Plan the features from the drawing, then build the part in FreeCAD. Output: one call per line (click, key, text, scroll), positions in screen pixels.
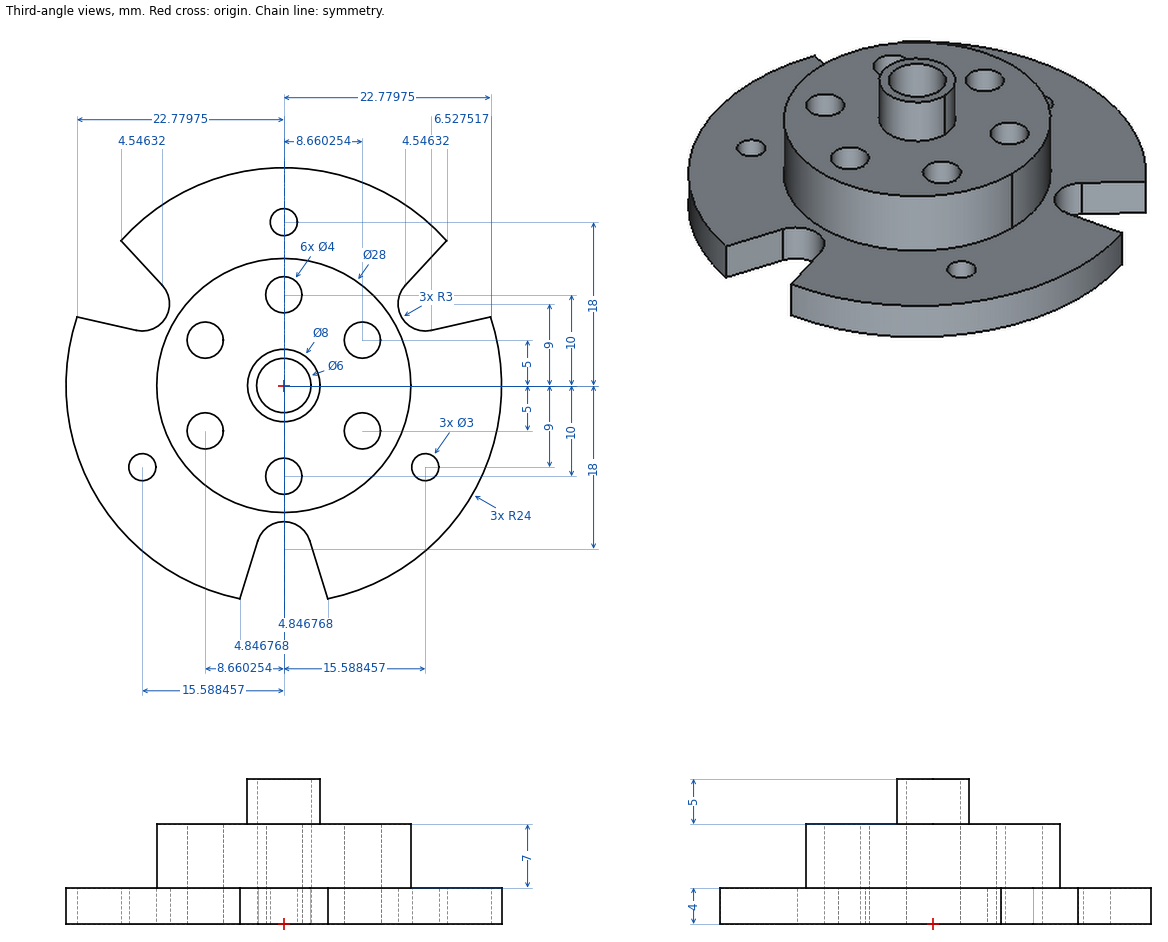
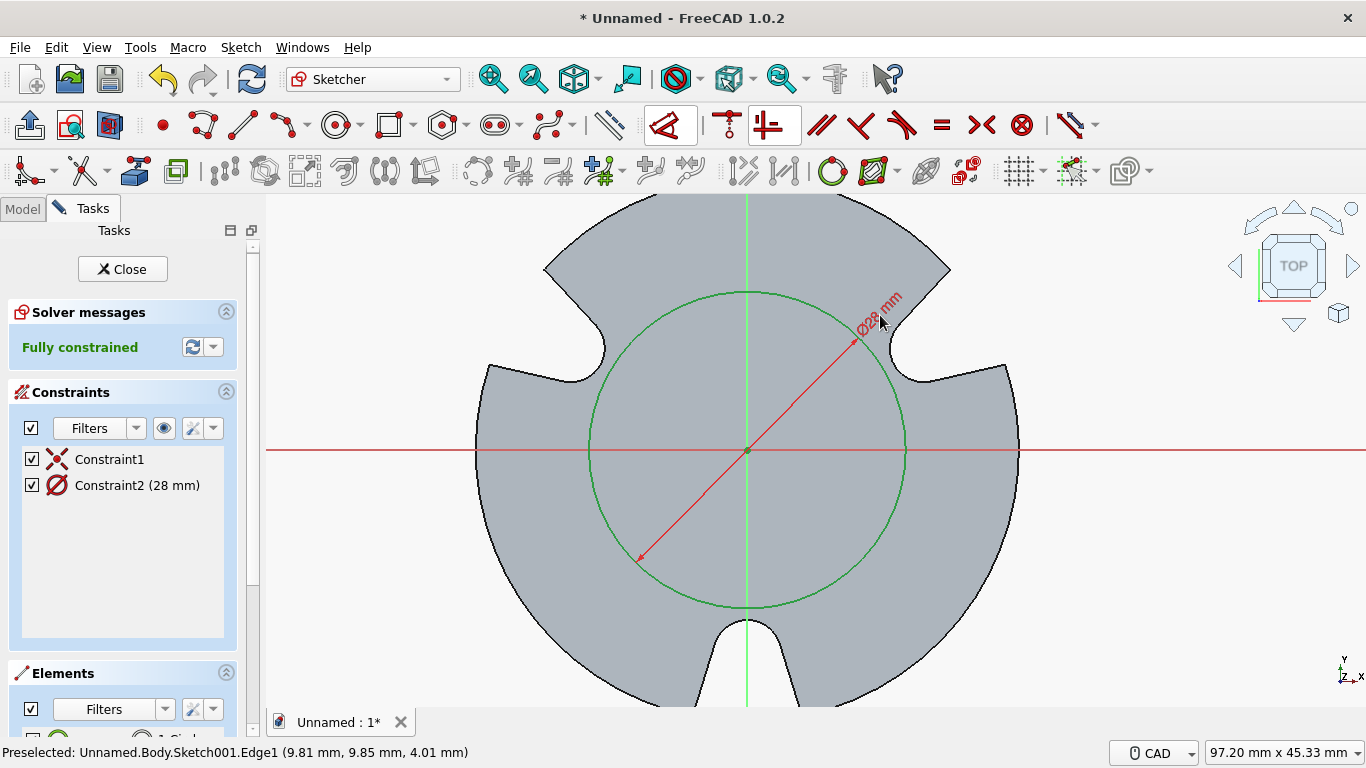
click(123, 269)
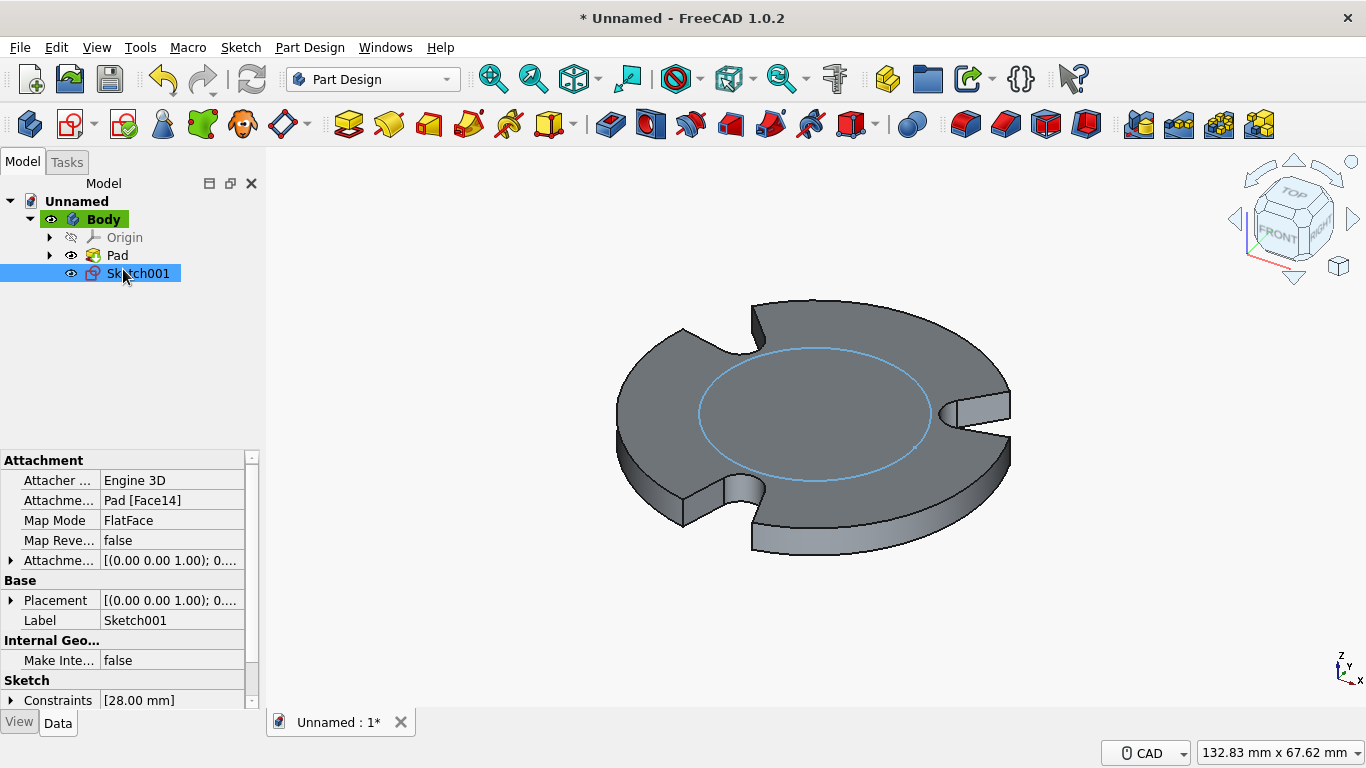
click(350, 124)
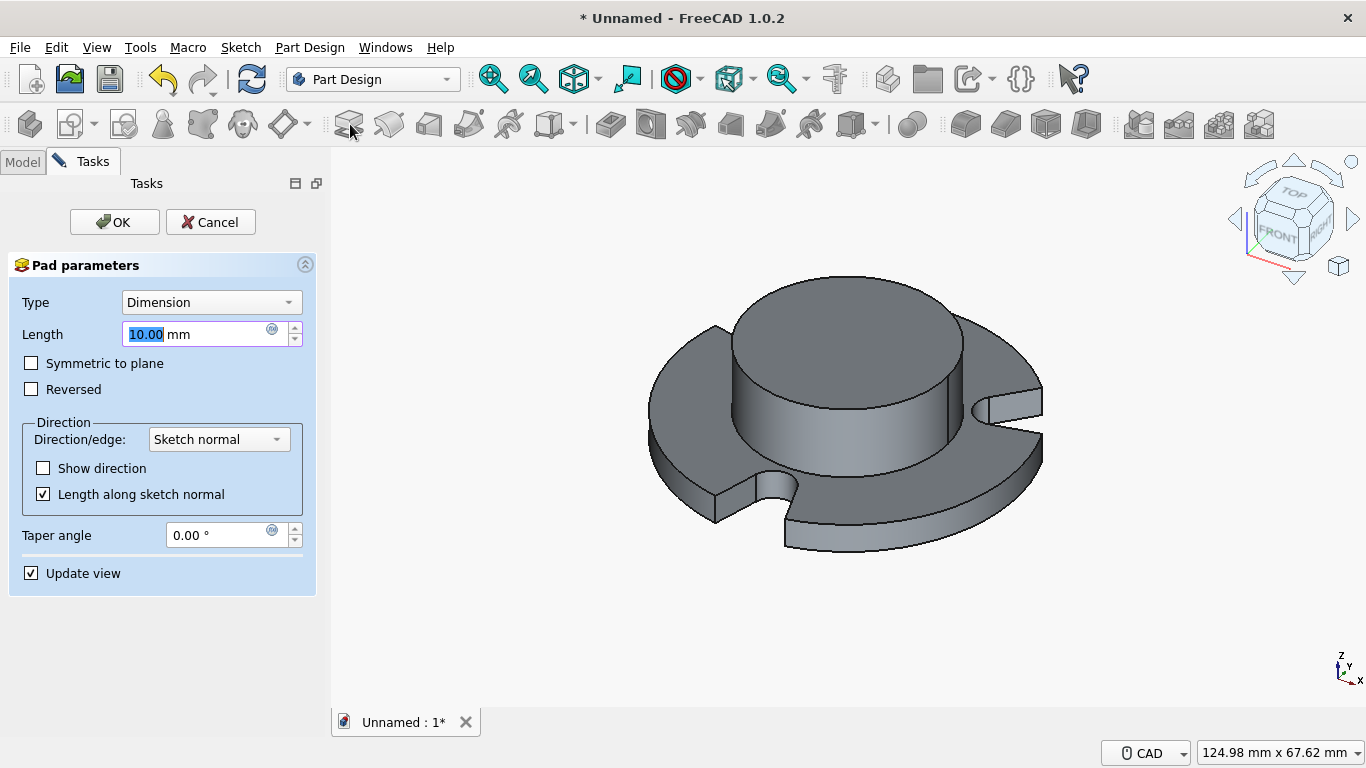
text(7)
key(Tab)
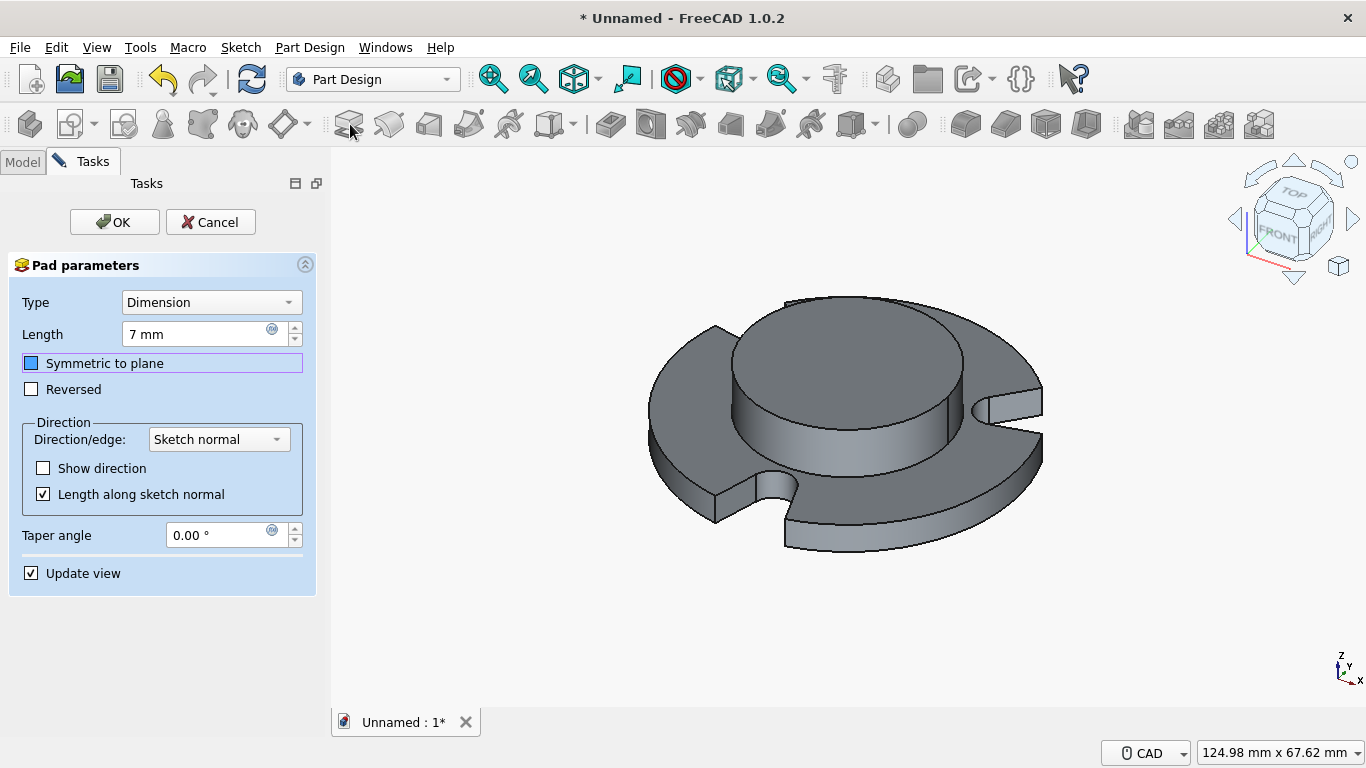
click(115, 222)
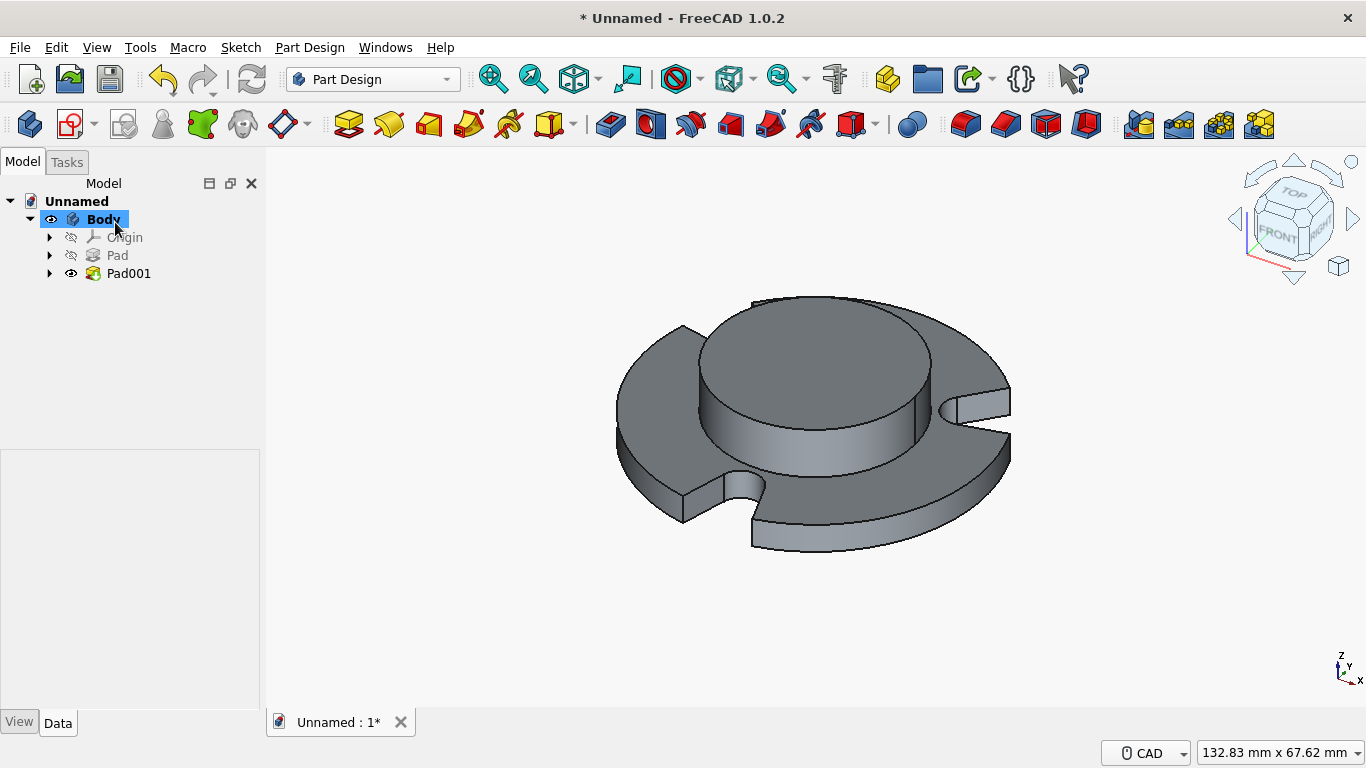
click(815, 362)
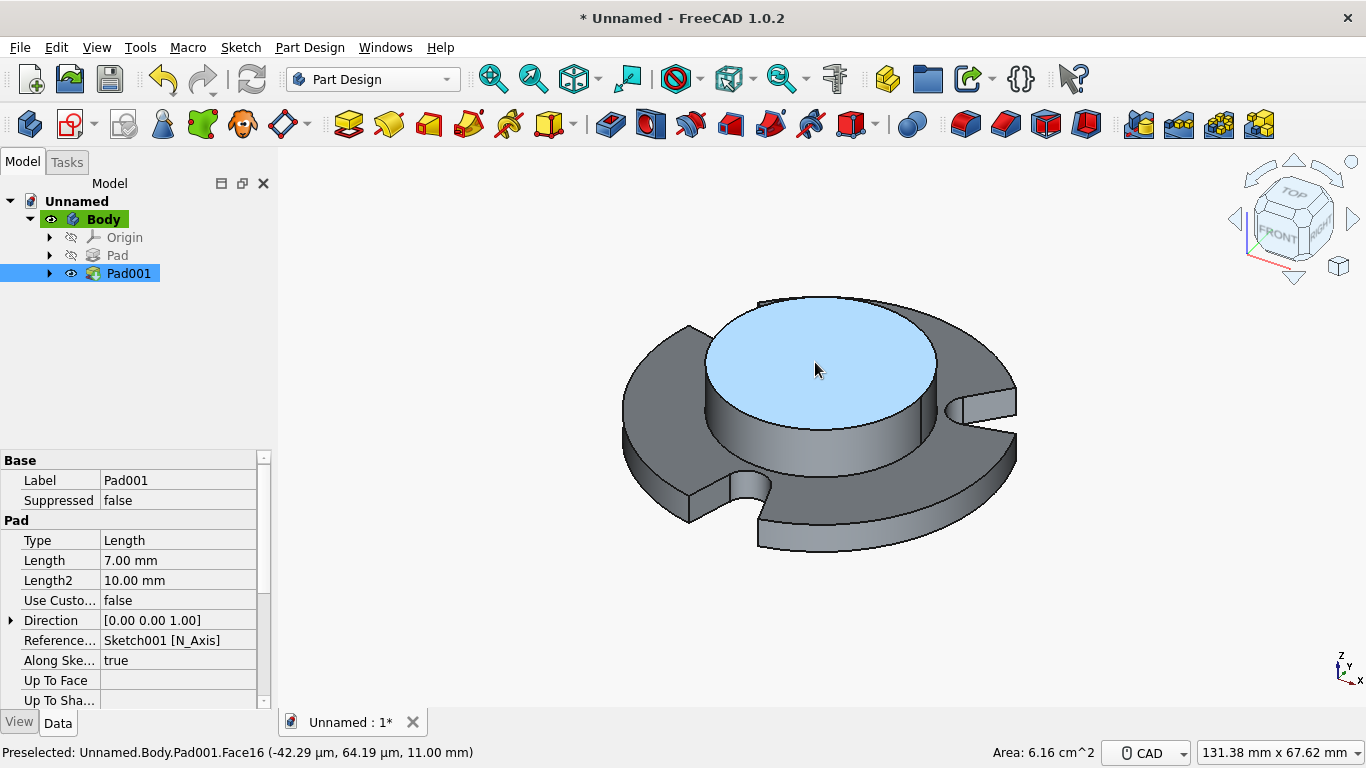
click(70, 124)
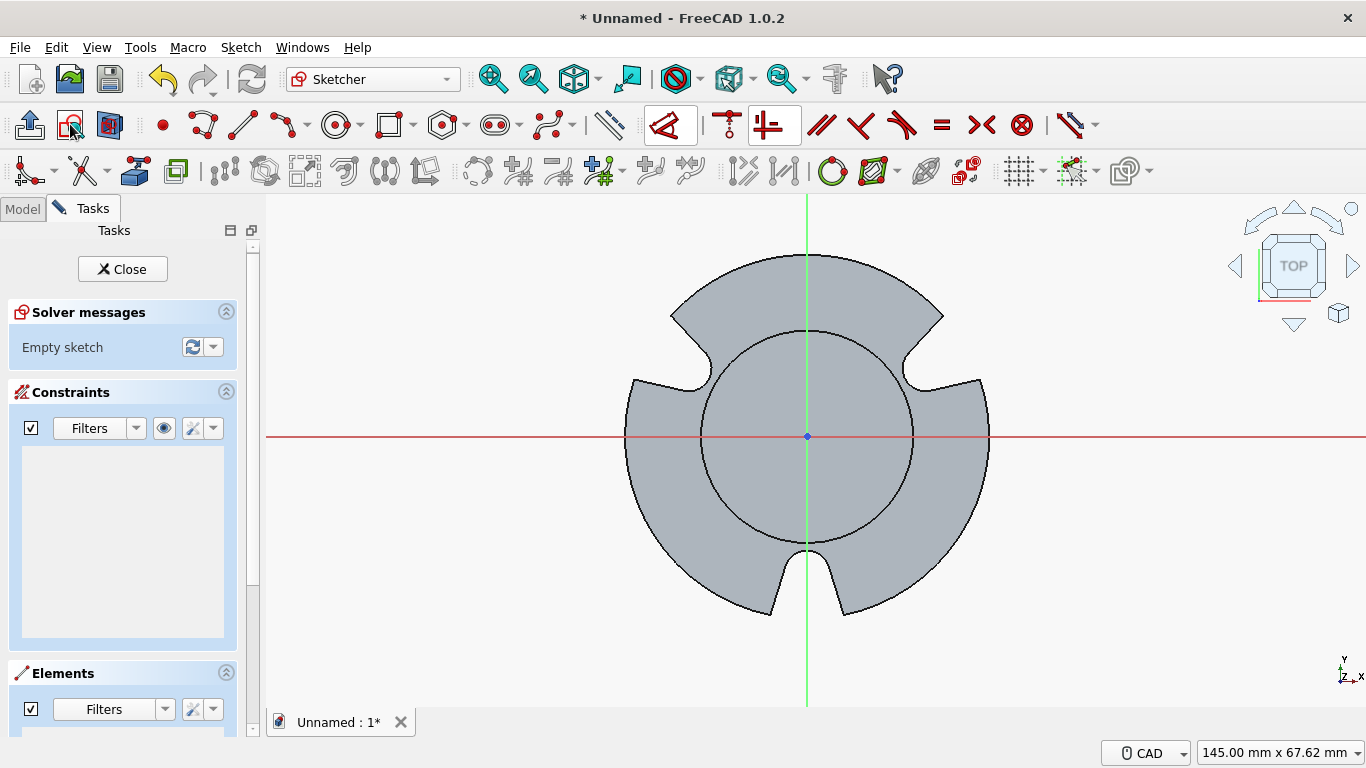
scroll(880, 420, up, 3)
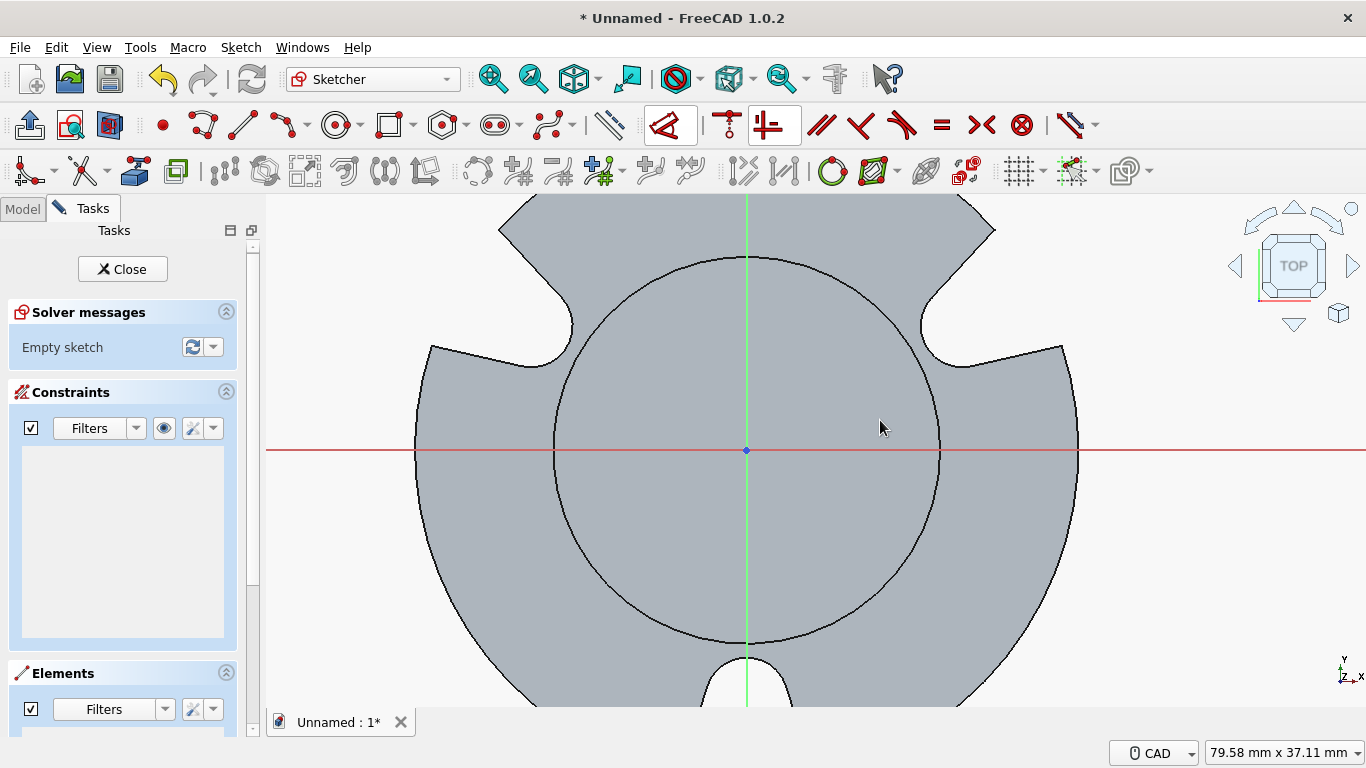
key(g)
key(c)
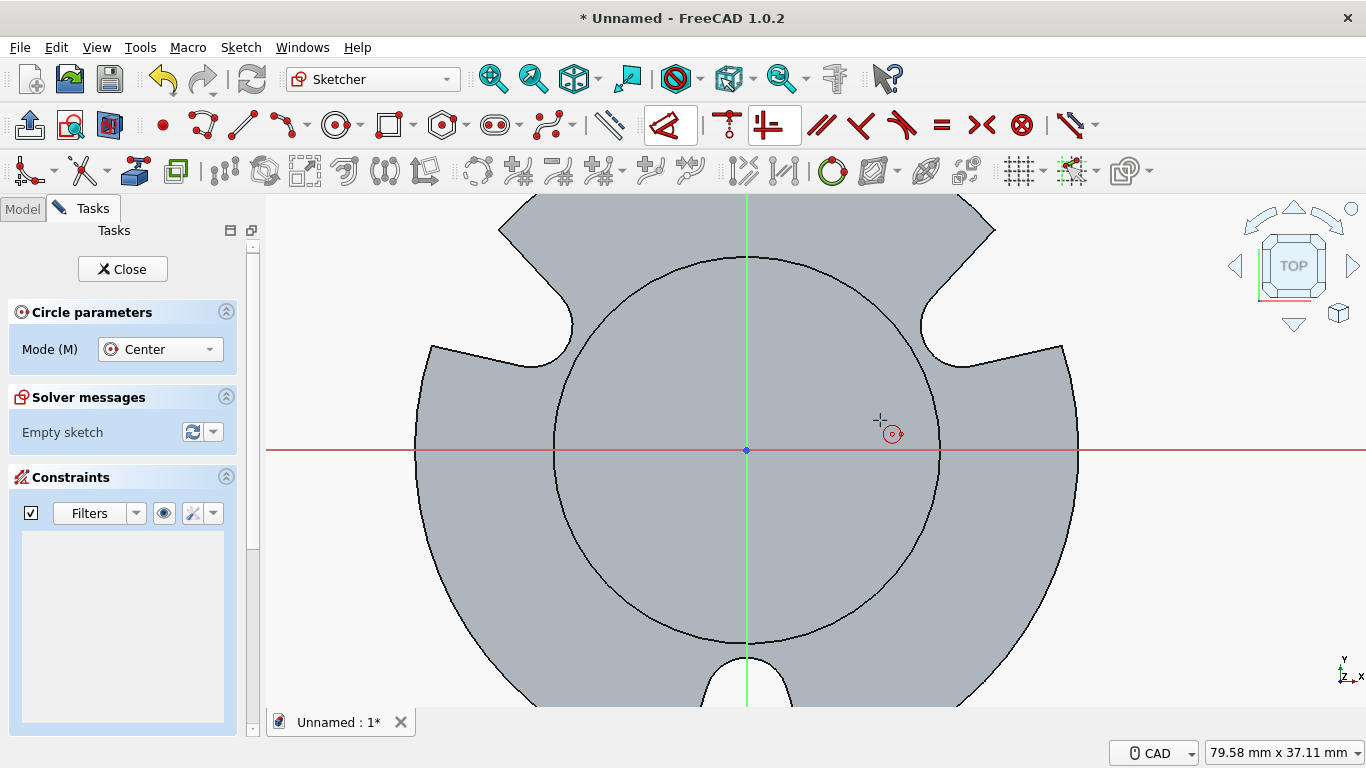
click(747, 312)
click(766, 293)